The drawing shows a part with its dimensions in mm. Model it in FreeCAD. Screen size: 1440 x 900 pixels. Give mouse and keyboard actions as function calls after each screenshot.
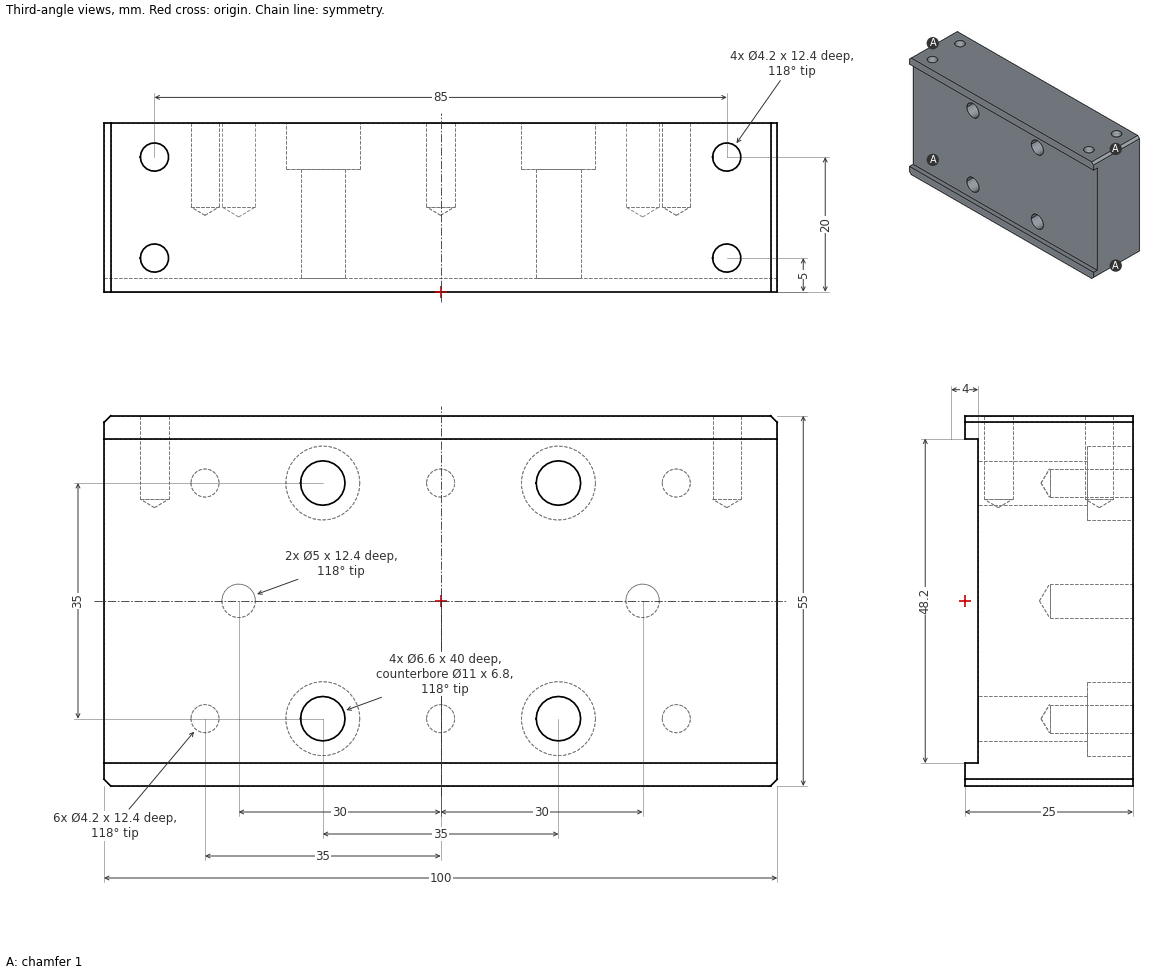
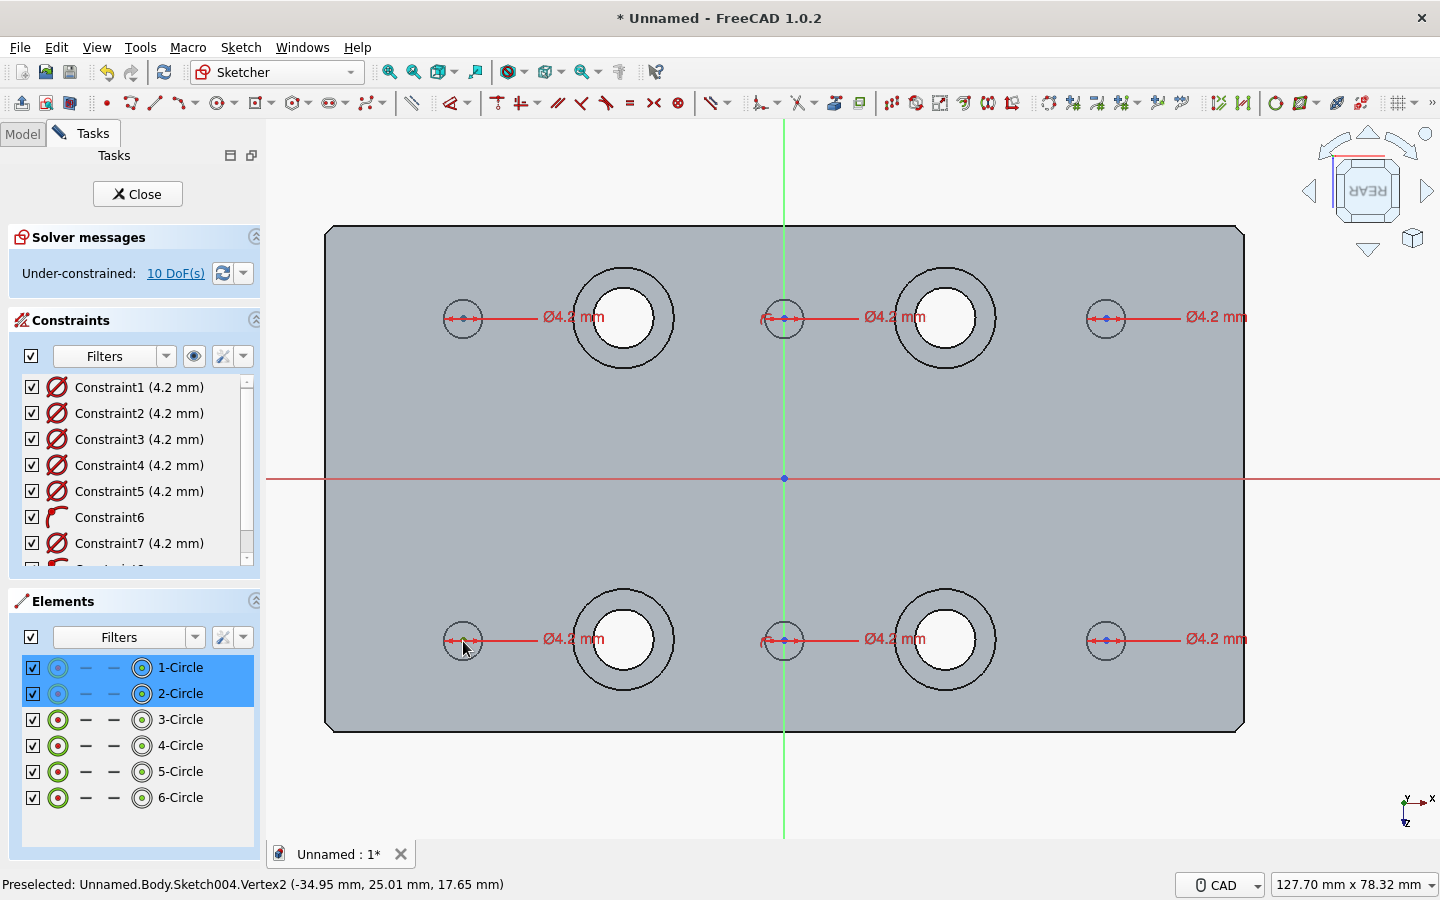
click(364, 479)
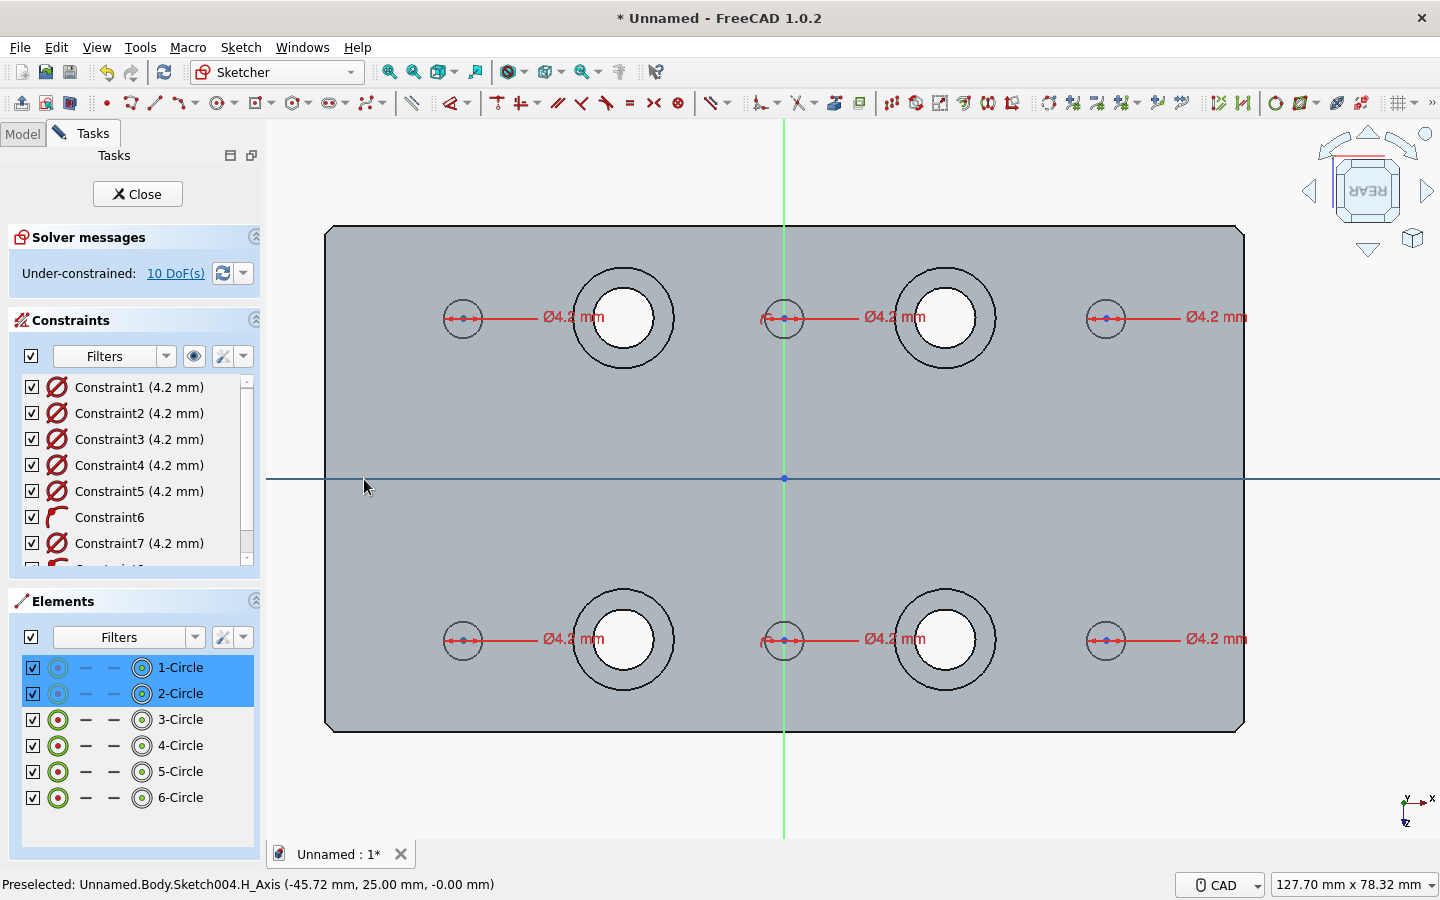
click(654, 104)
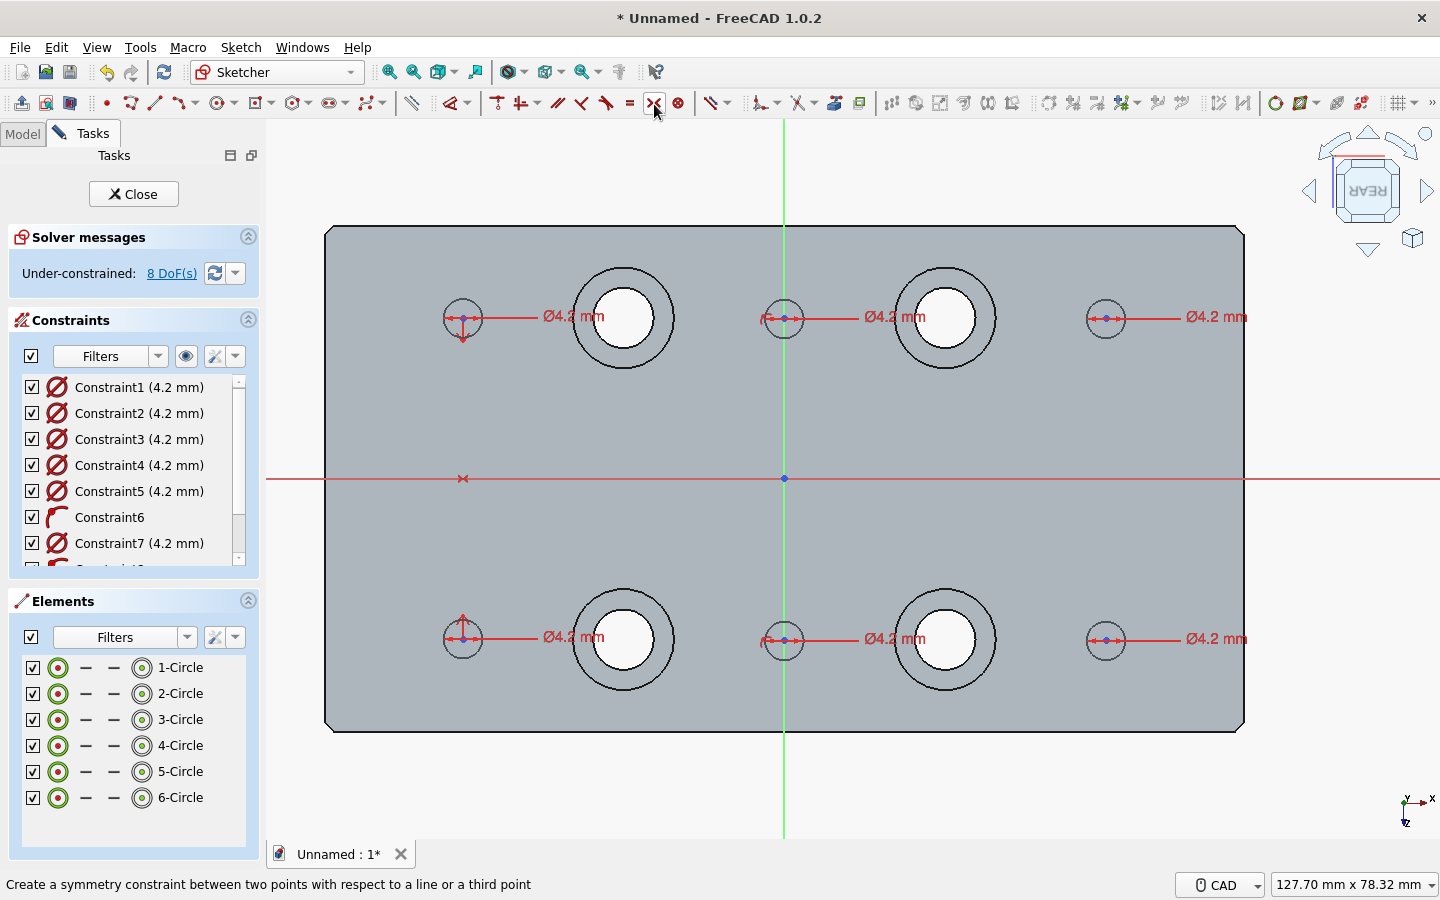
click(463, 318)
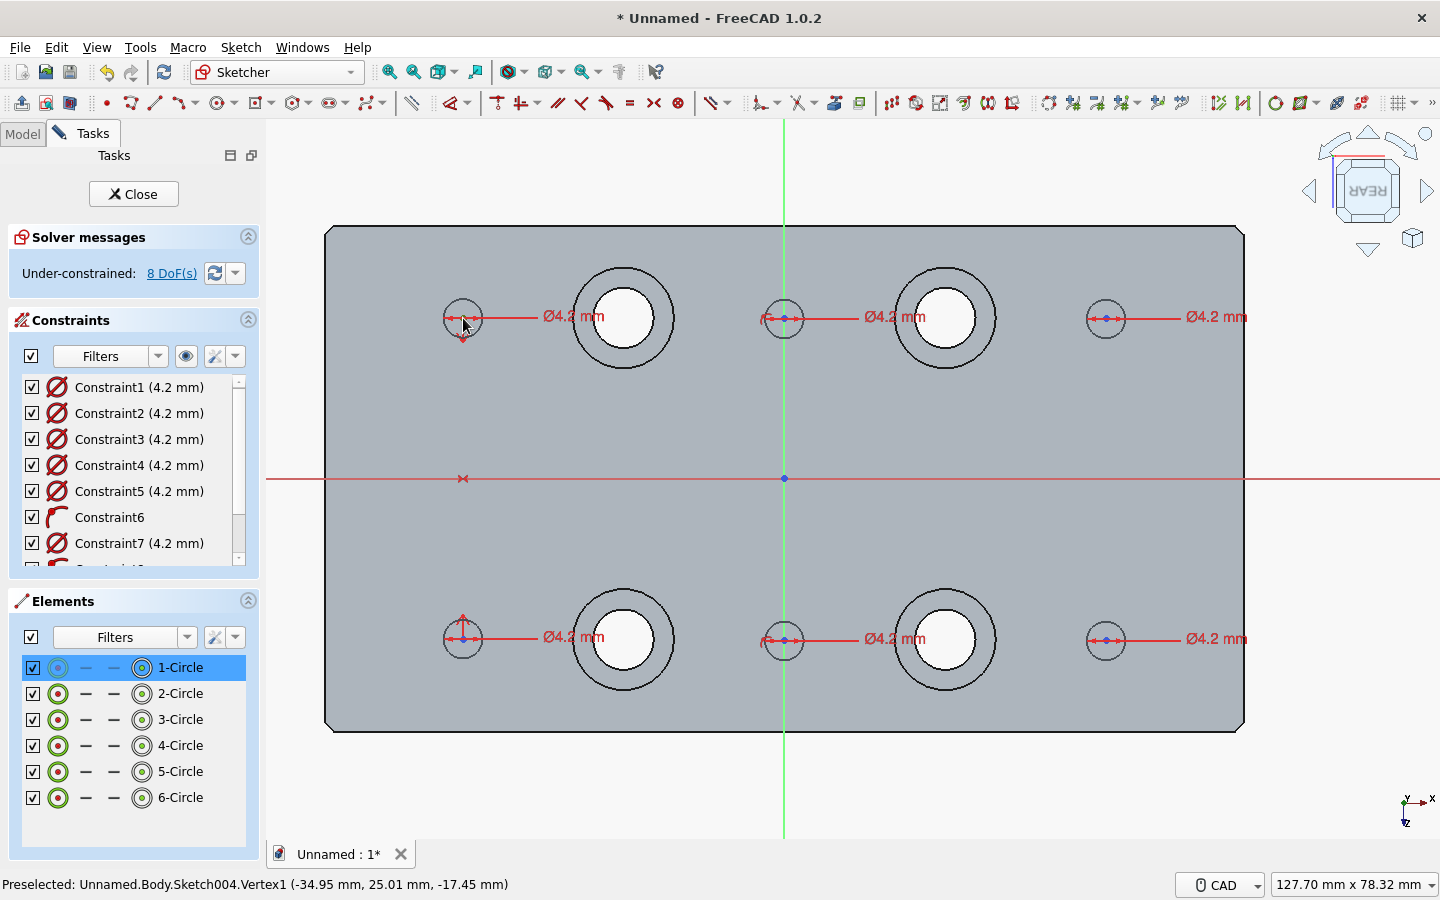
click(1106, 319)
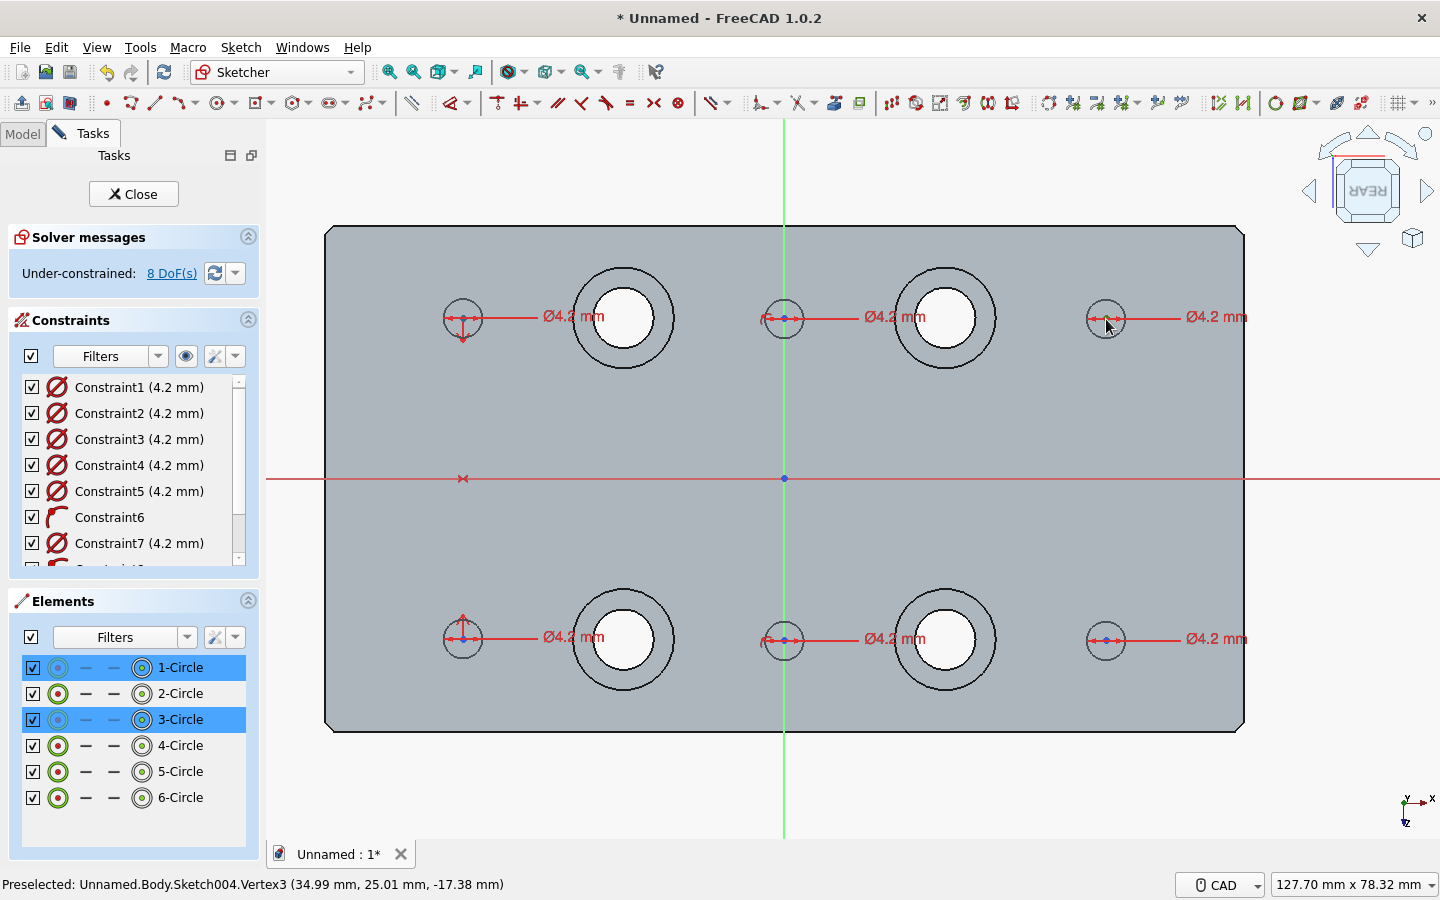
click(784, 764)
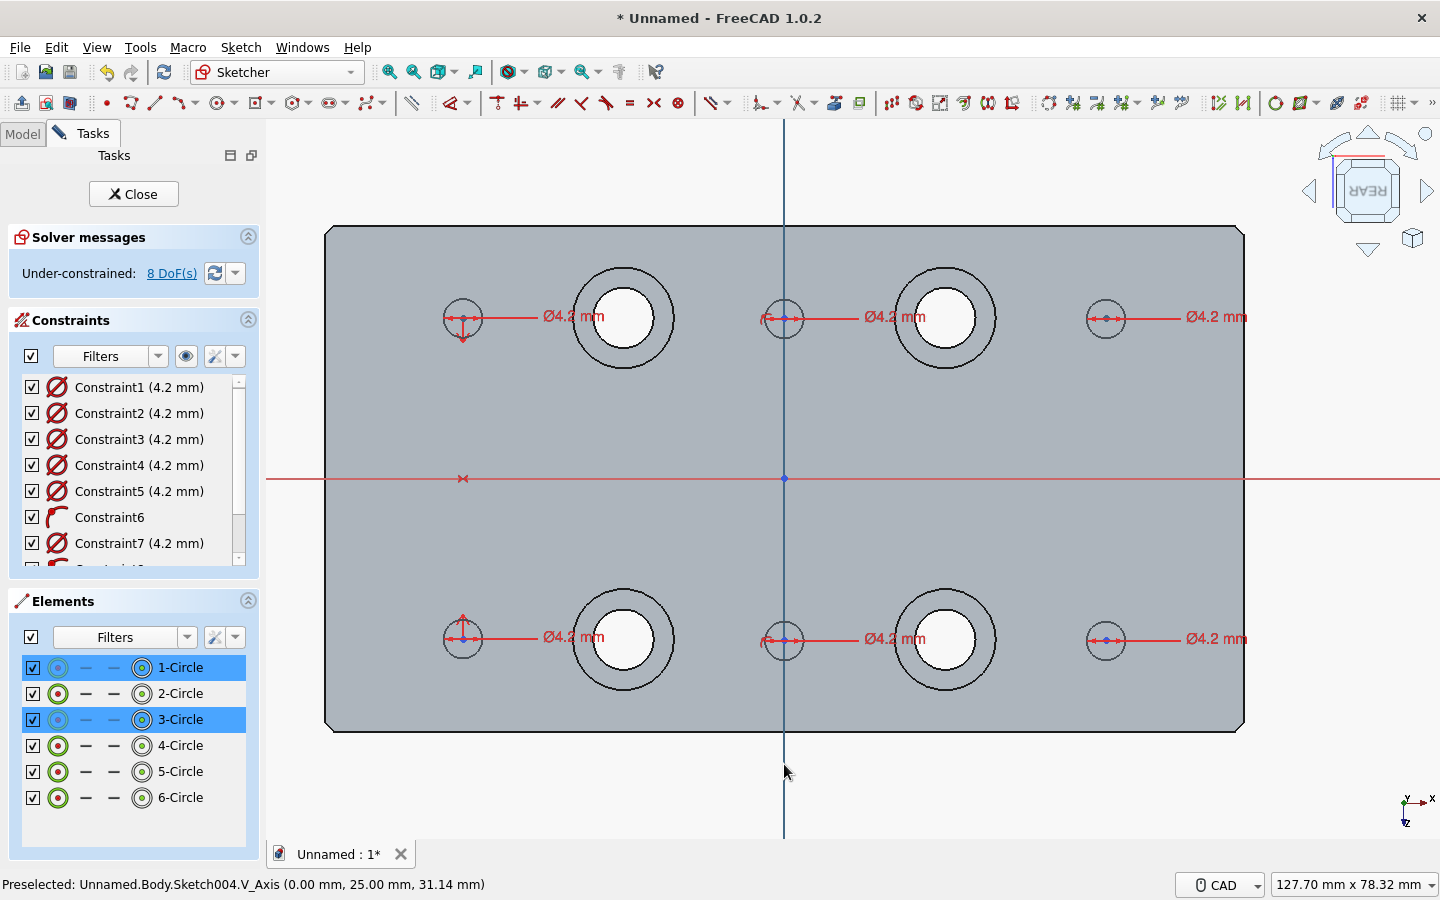
click(654, 104)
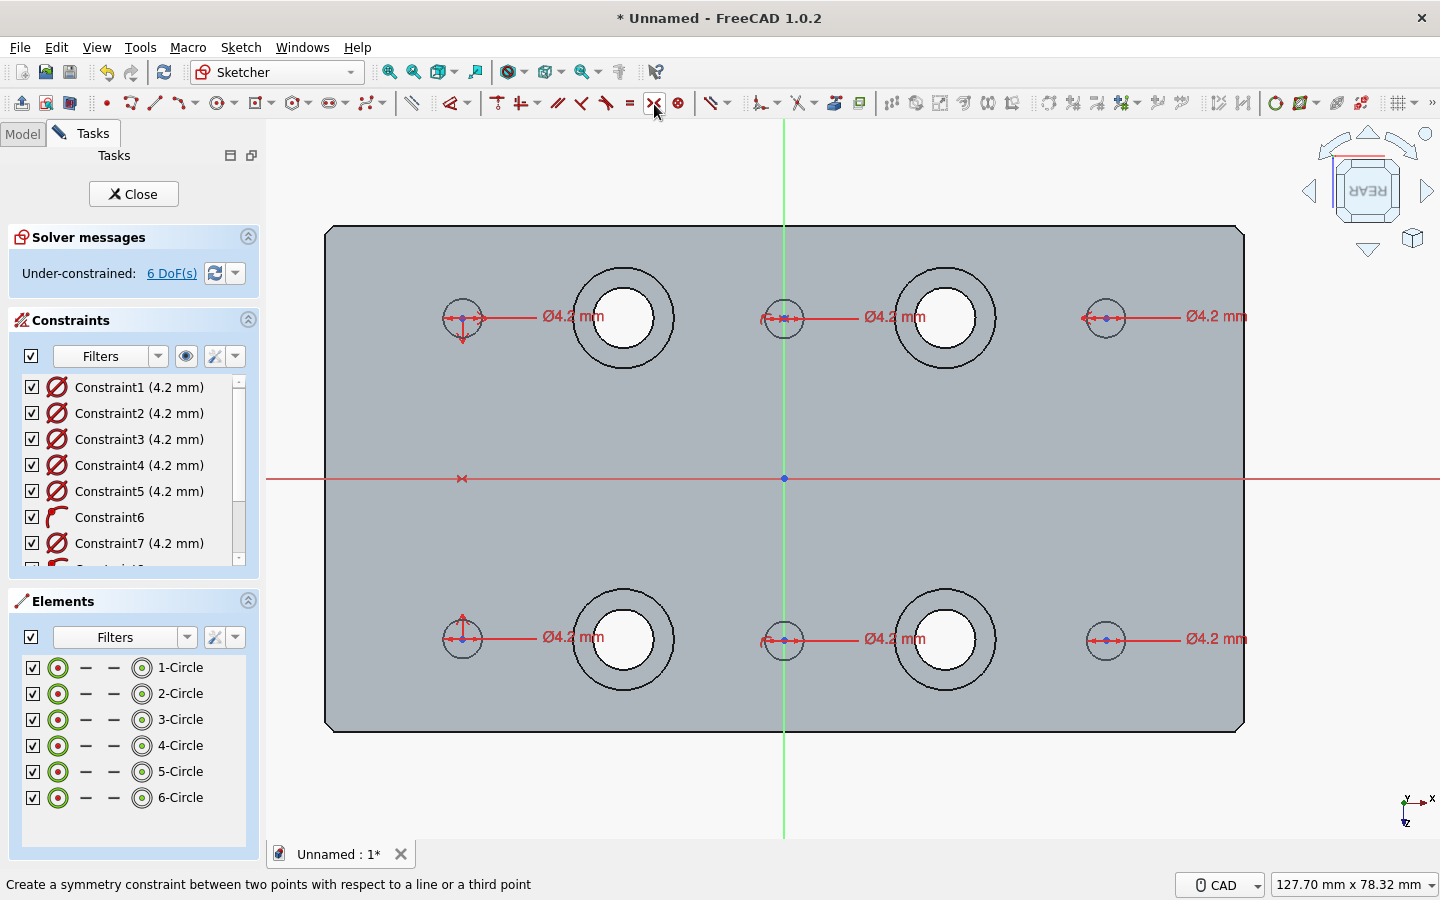
click(463, 639)